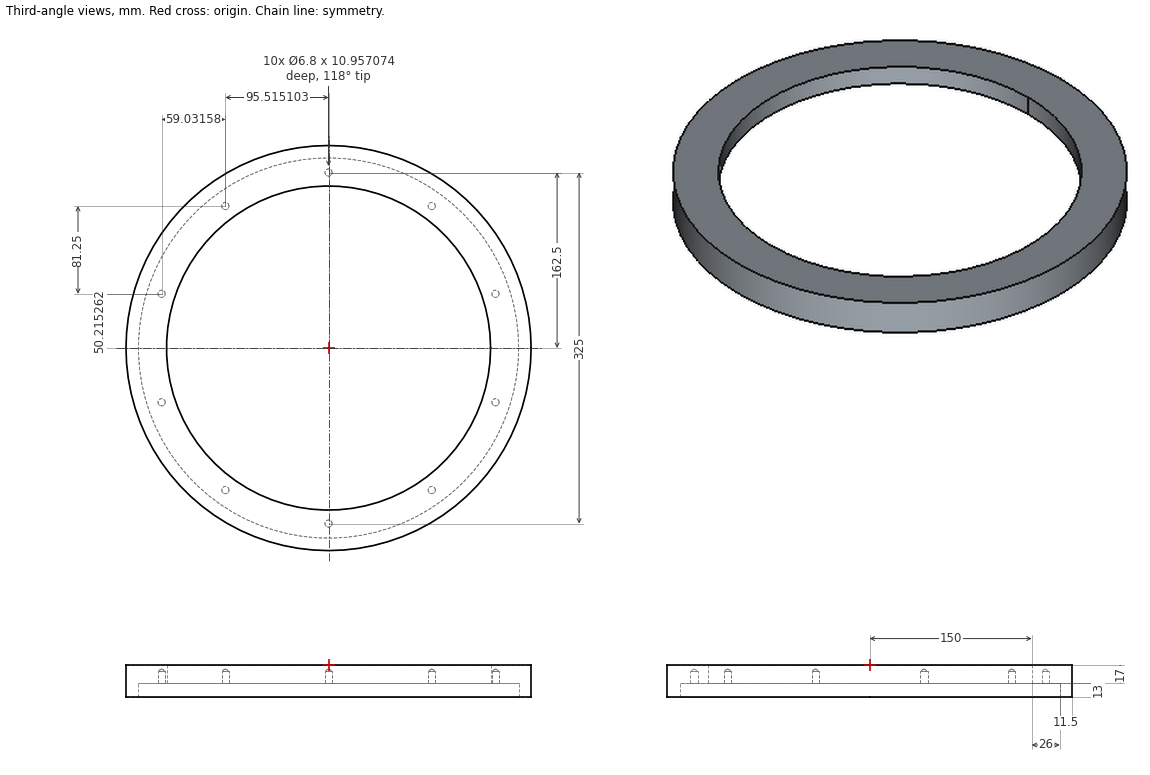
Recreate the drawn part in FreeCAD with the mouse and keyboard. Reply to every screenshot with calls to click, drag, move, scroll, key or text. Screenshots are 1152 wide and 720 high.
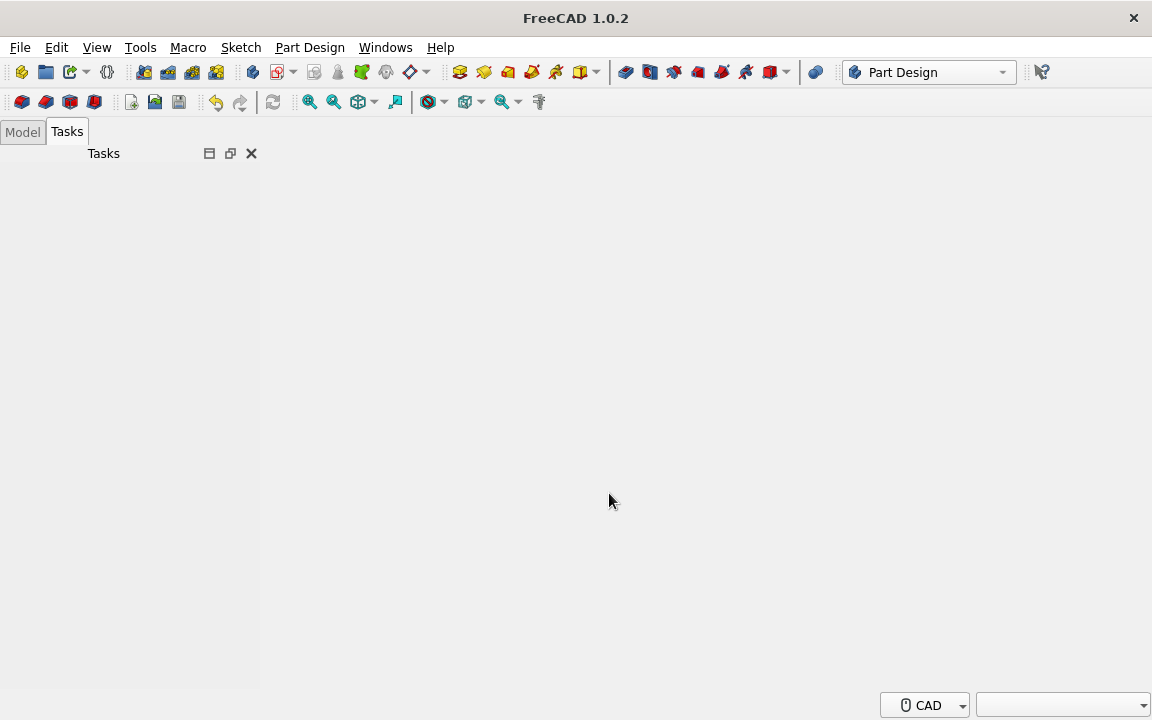
click(132, 102)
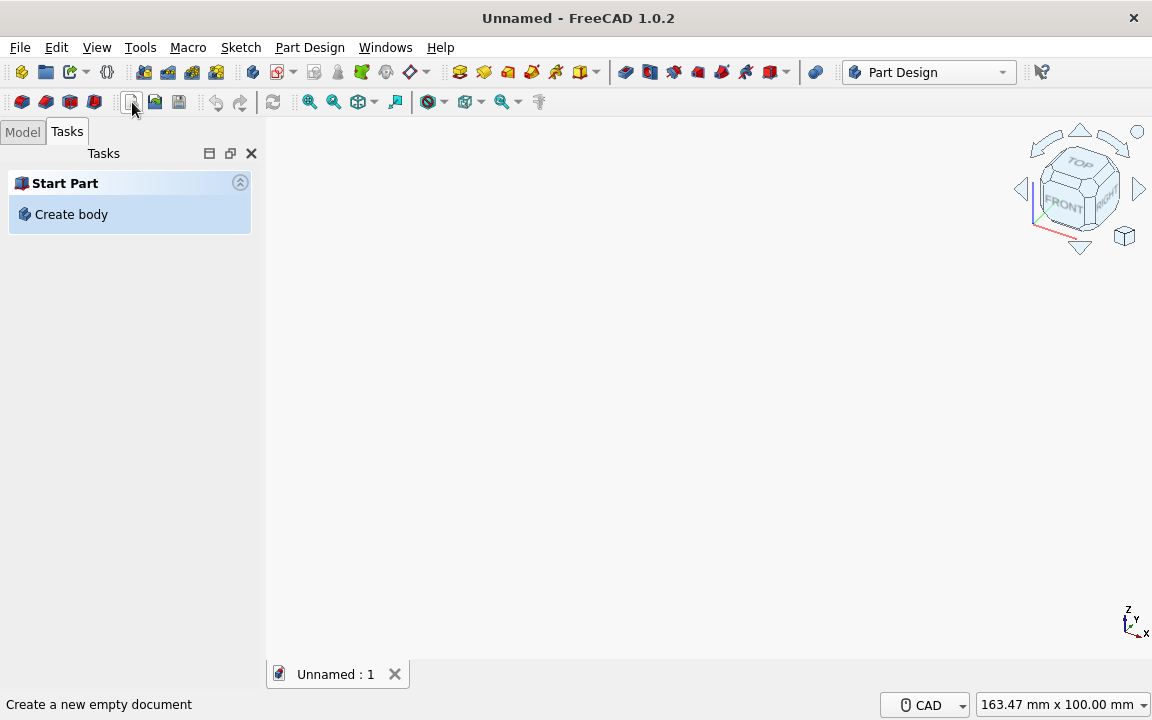
click(278, 72)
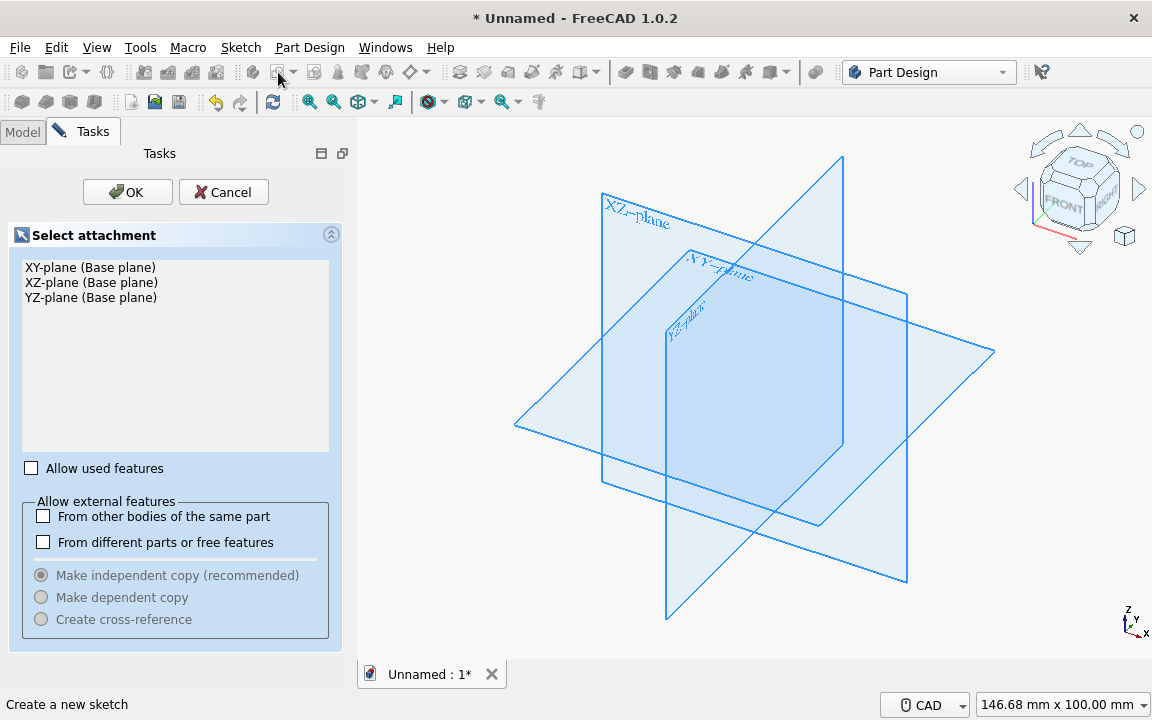
click(82, 298)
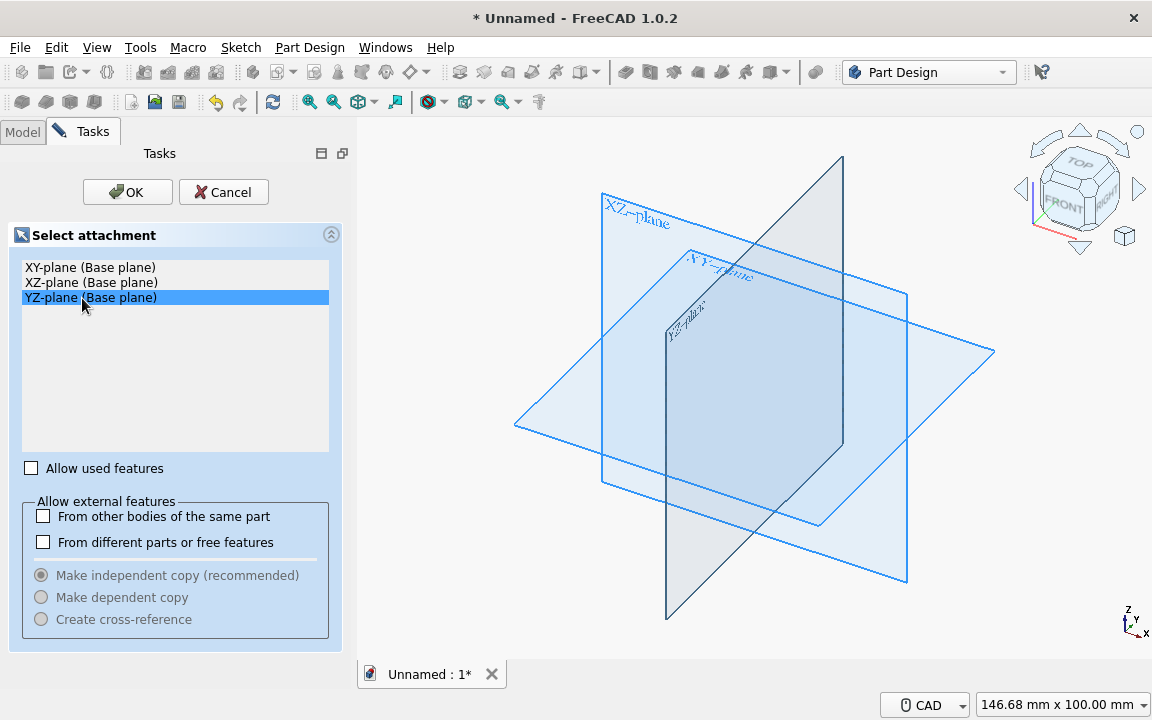
click(128, 192)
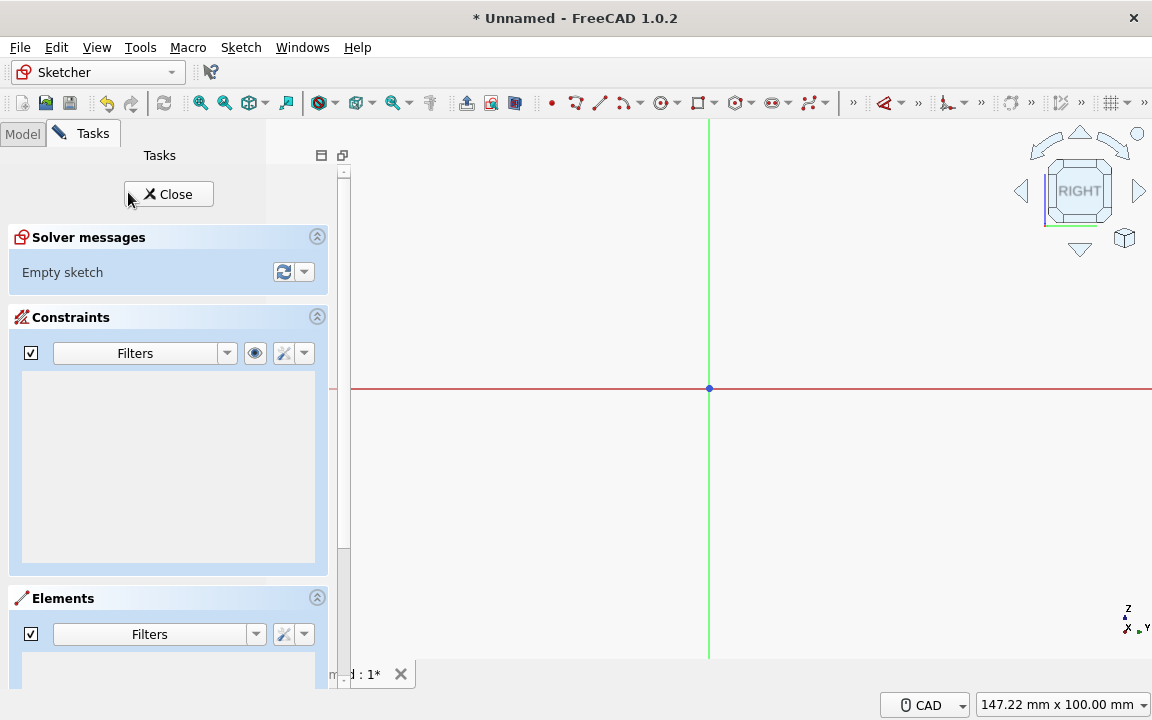
scroll(640, 389, down, 5)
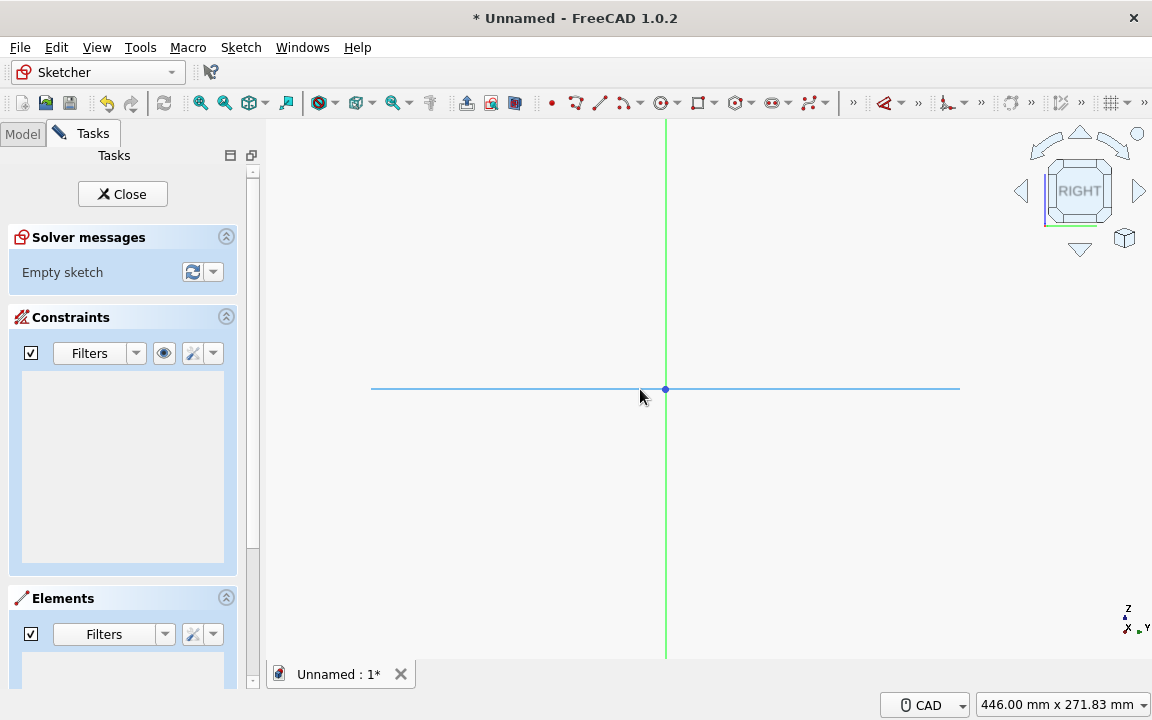
scroll(640, 389, down, 5)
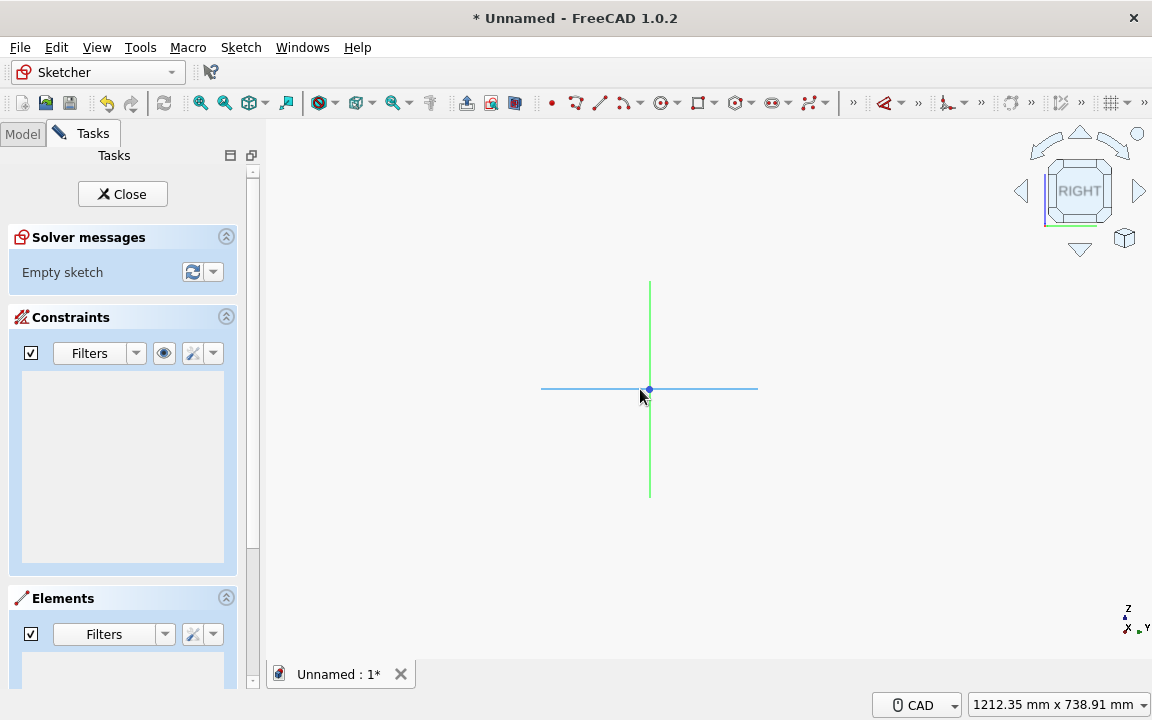
scroll(782, 401, up, 14)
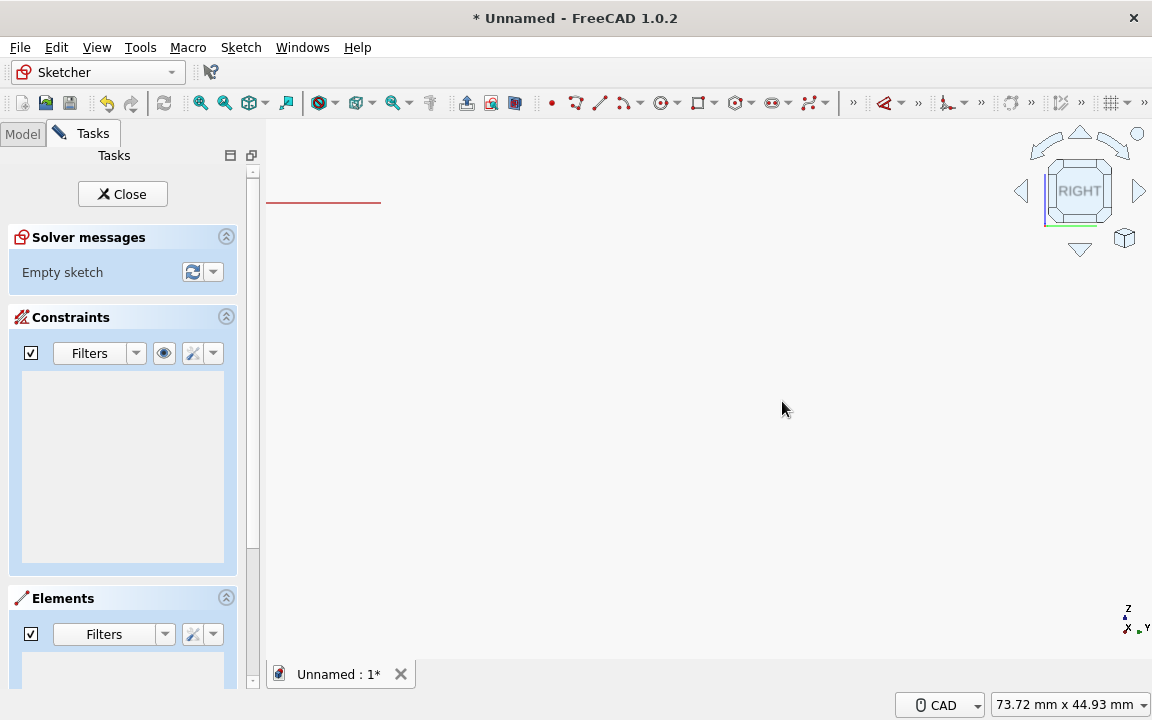
key(g)
key(m)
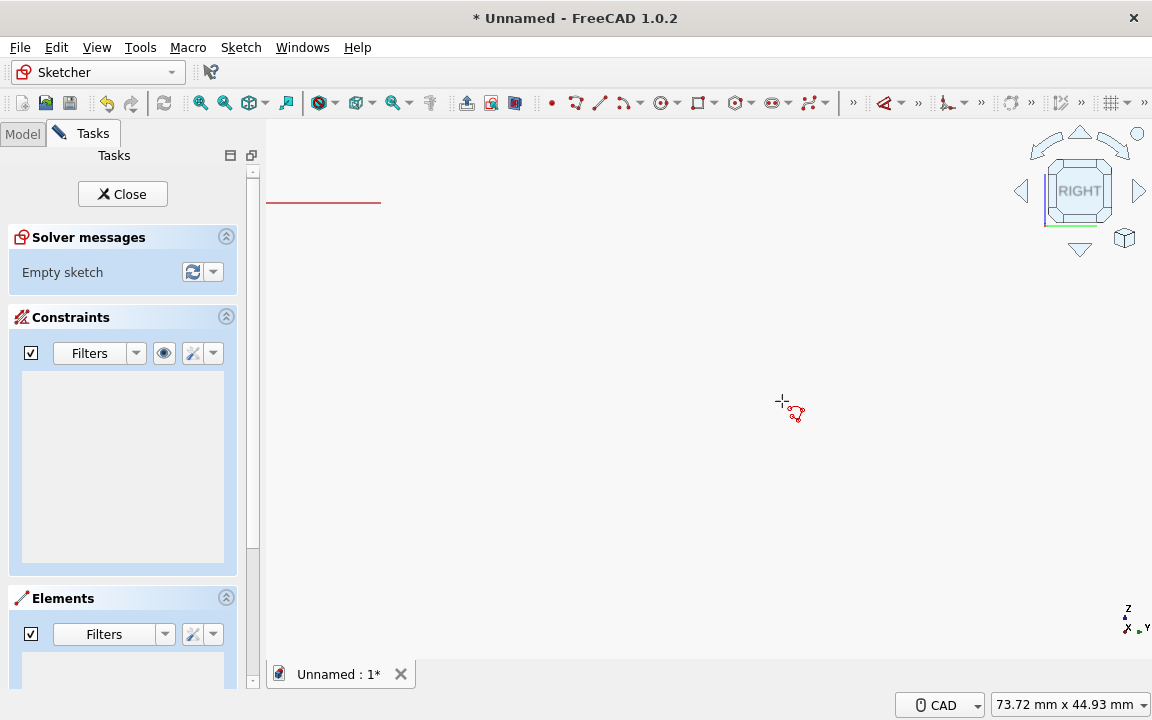
click(400, 203)
click(400, 407)
click(713, 407)
click(713, 563)
click(851, 563)
click(851, 212)
click(400, 204)
key(Escape)
key(Escape)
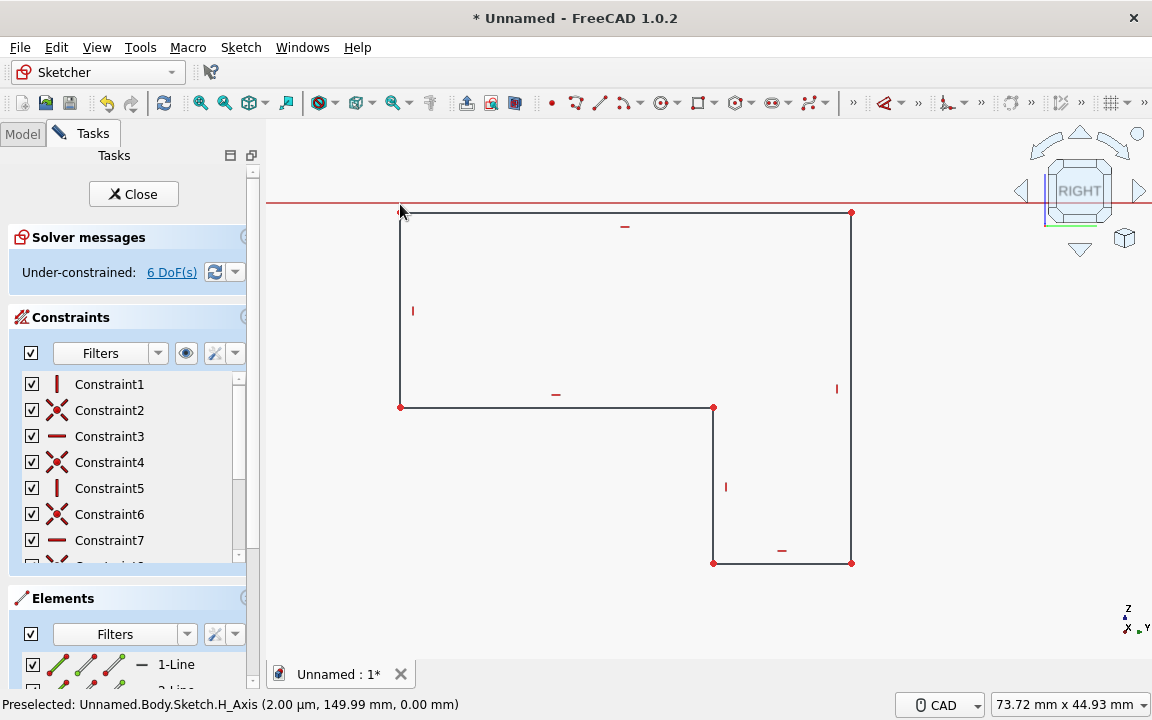
click(400, 213)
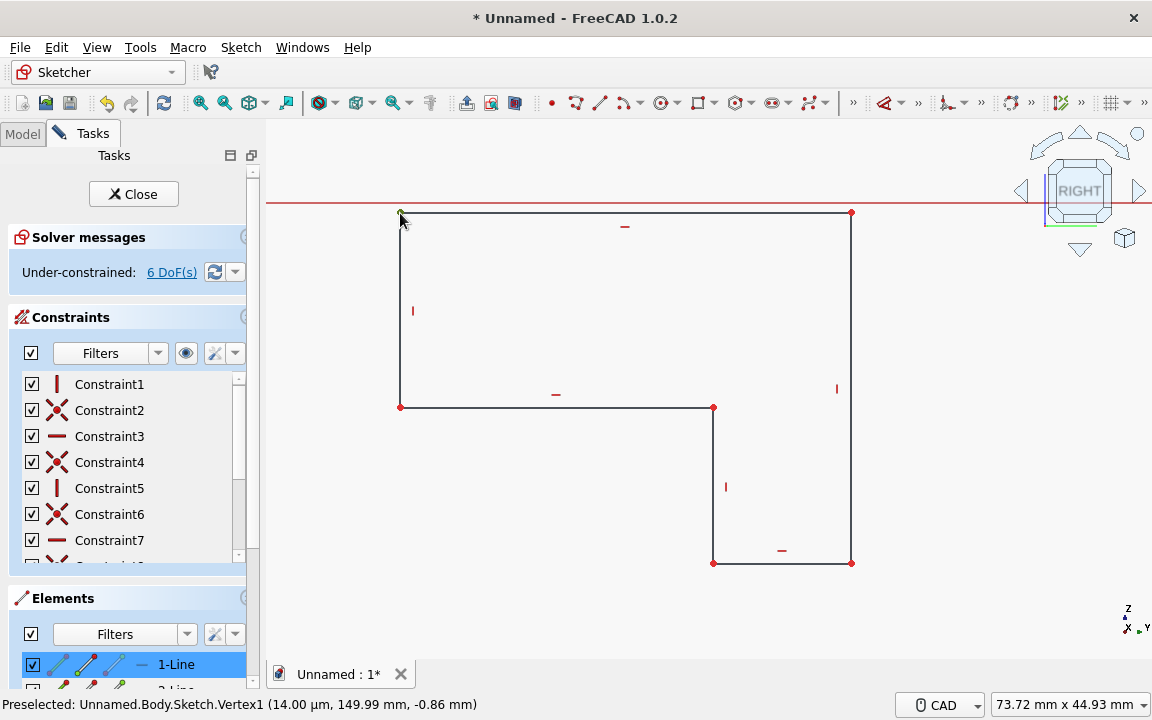
click(344, 203)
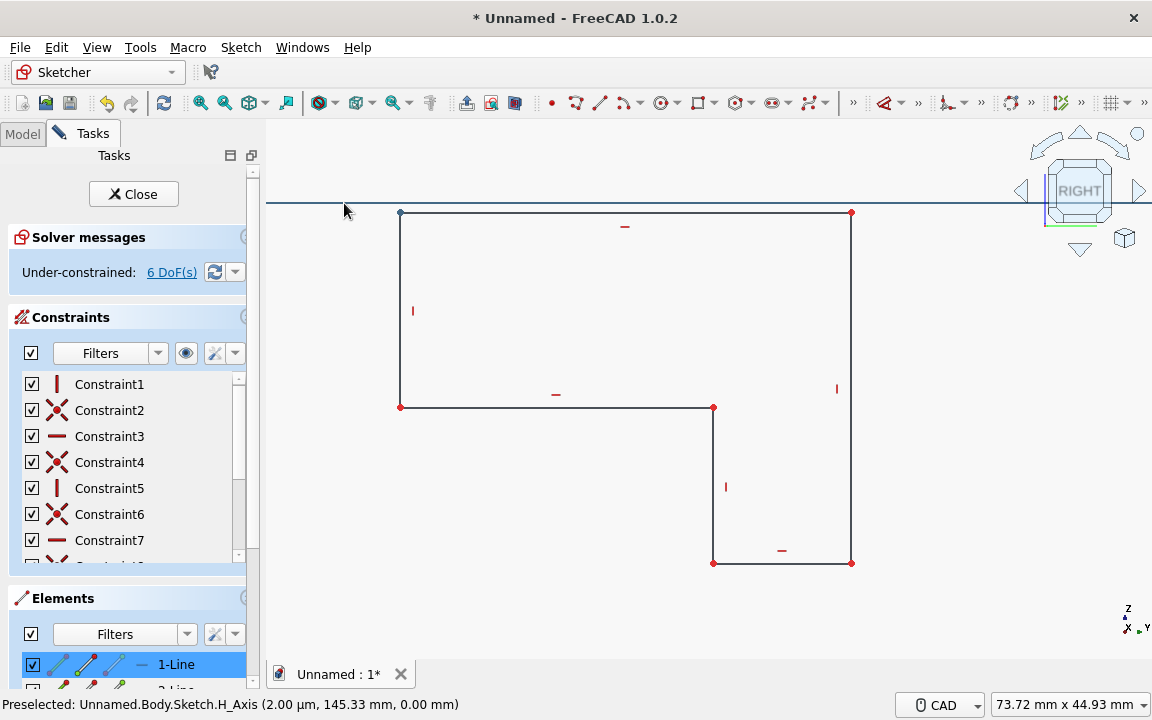
key(c)